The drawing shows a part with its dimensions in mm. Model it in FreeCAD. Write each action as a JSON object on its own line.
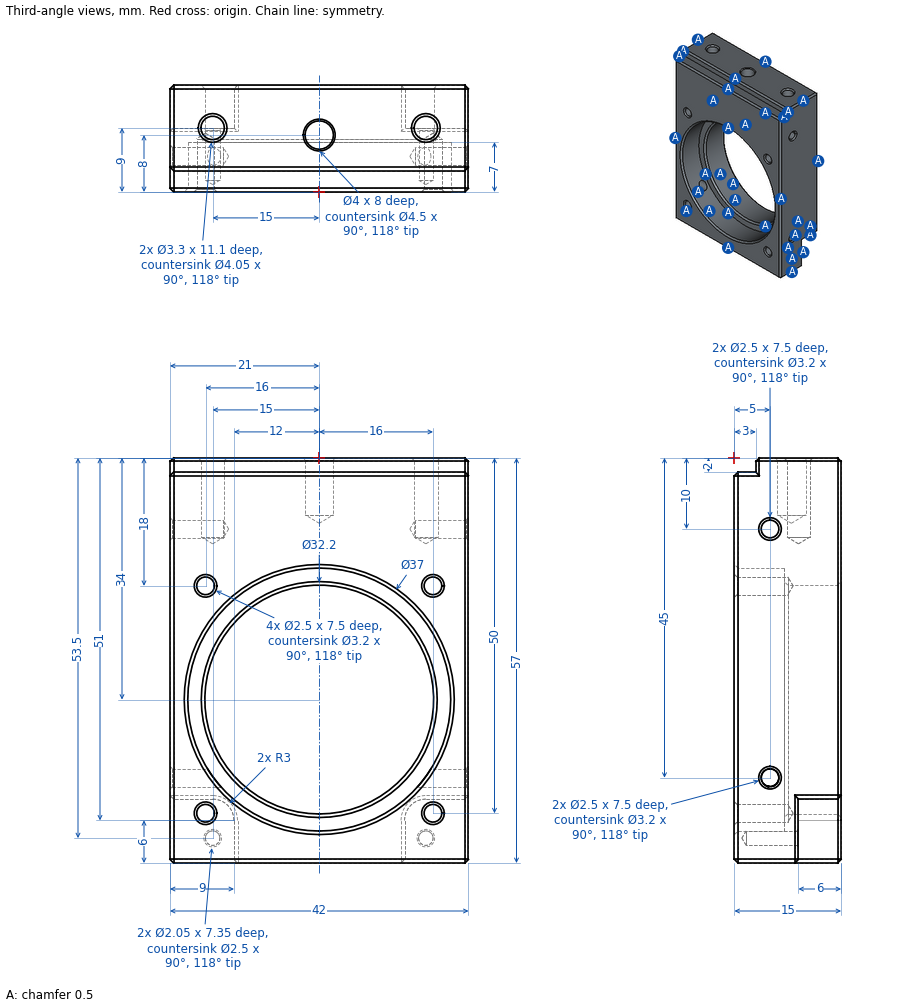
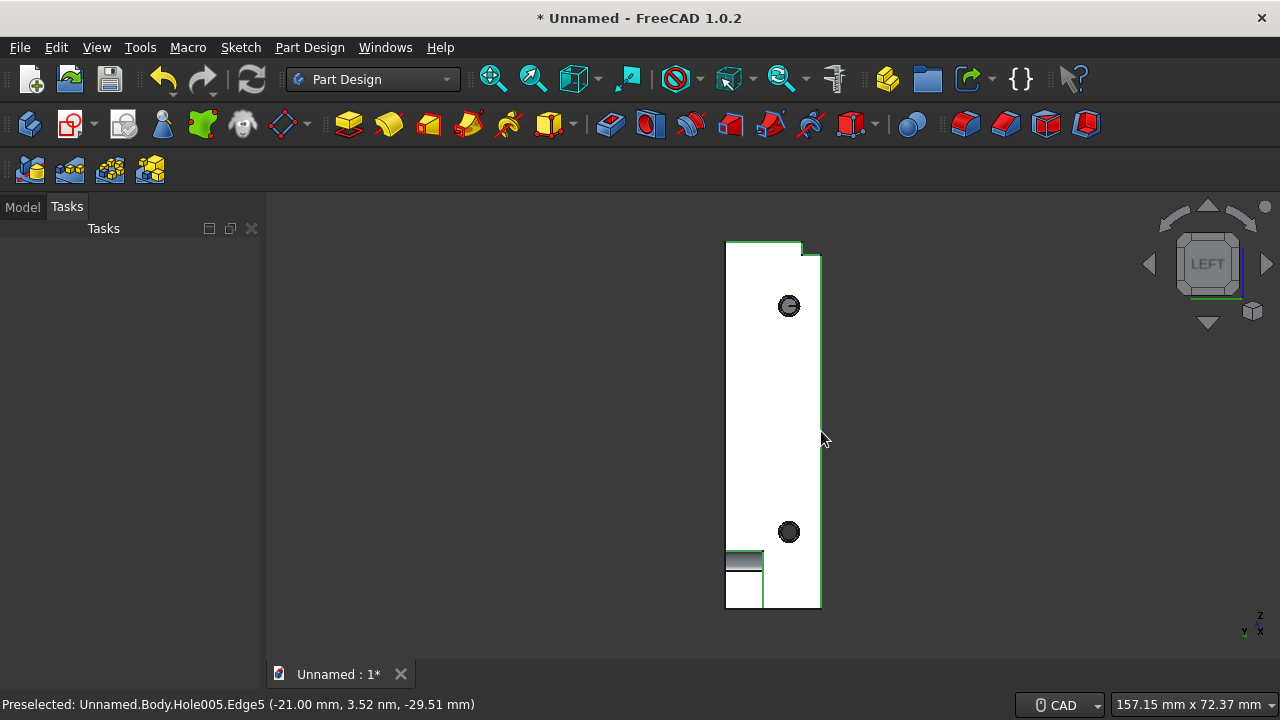
{"action": "left_click", "coordinate": [1006, 124]}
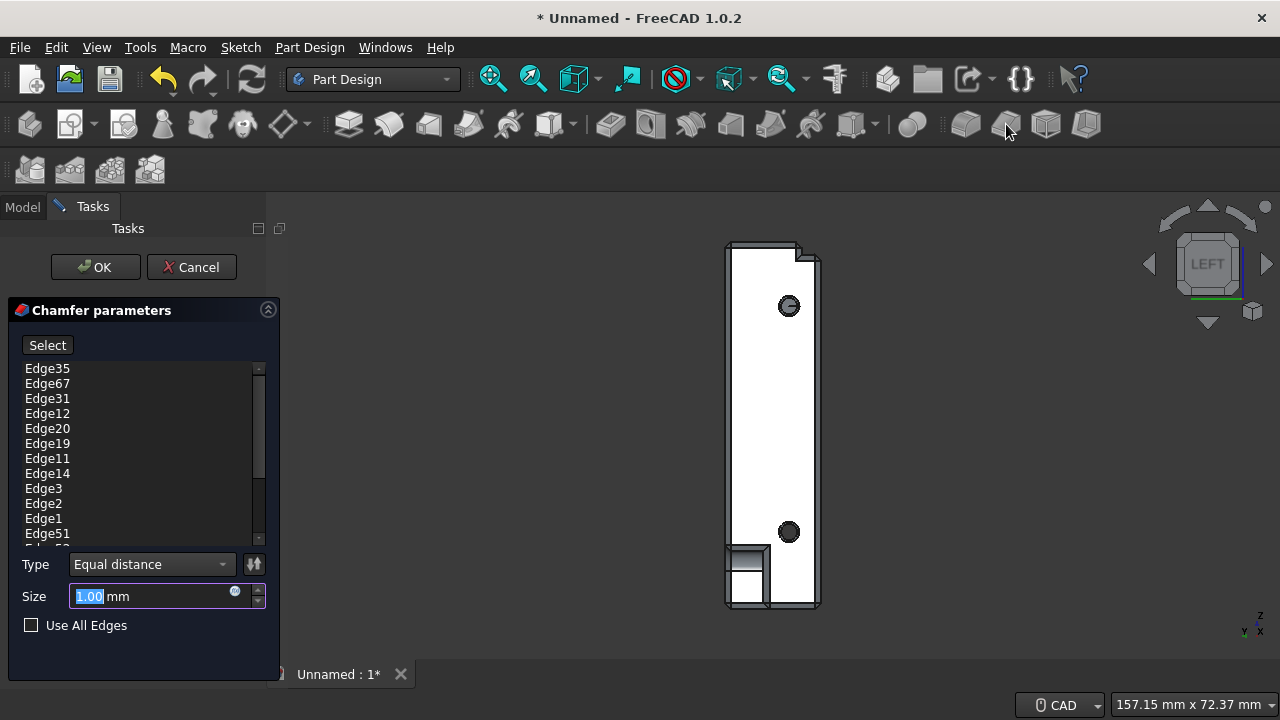
{"action": "type", "text": "0.5"}
{"action": "key", "text": "Tab"}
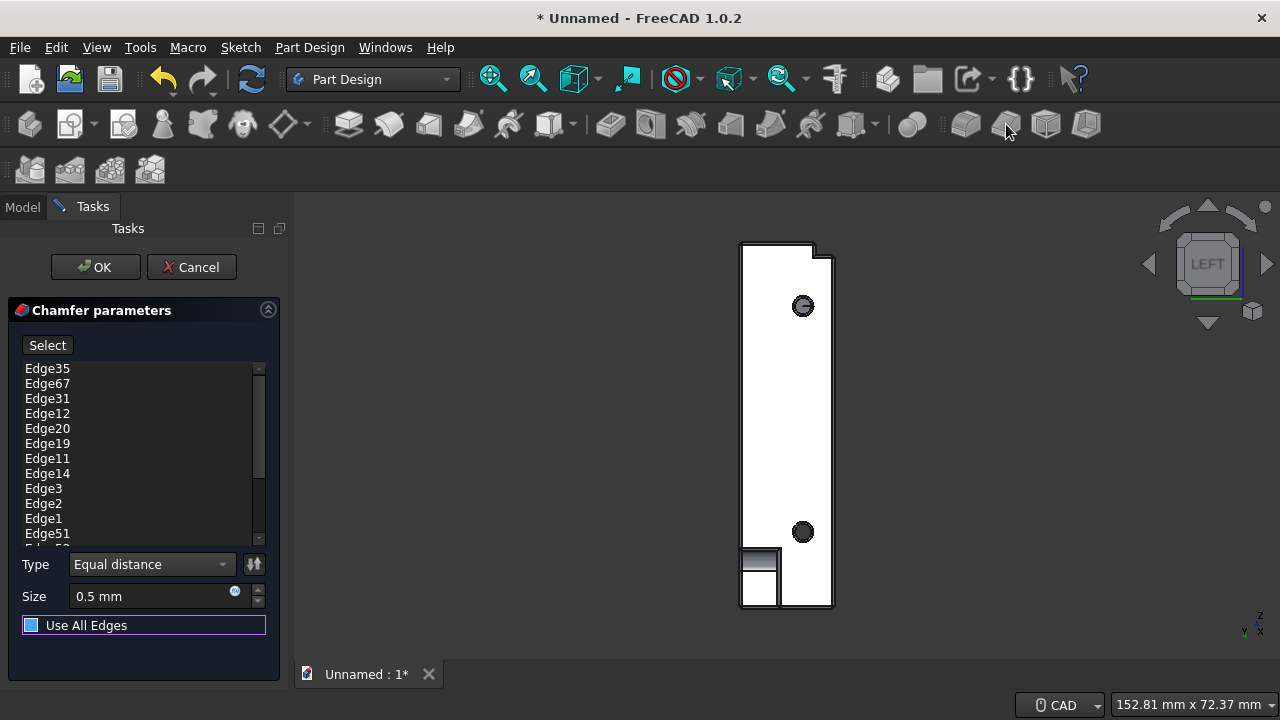
{"action": "left_click", "coordinate": [96, 267]}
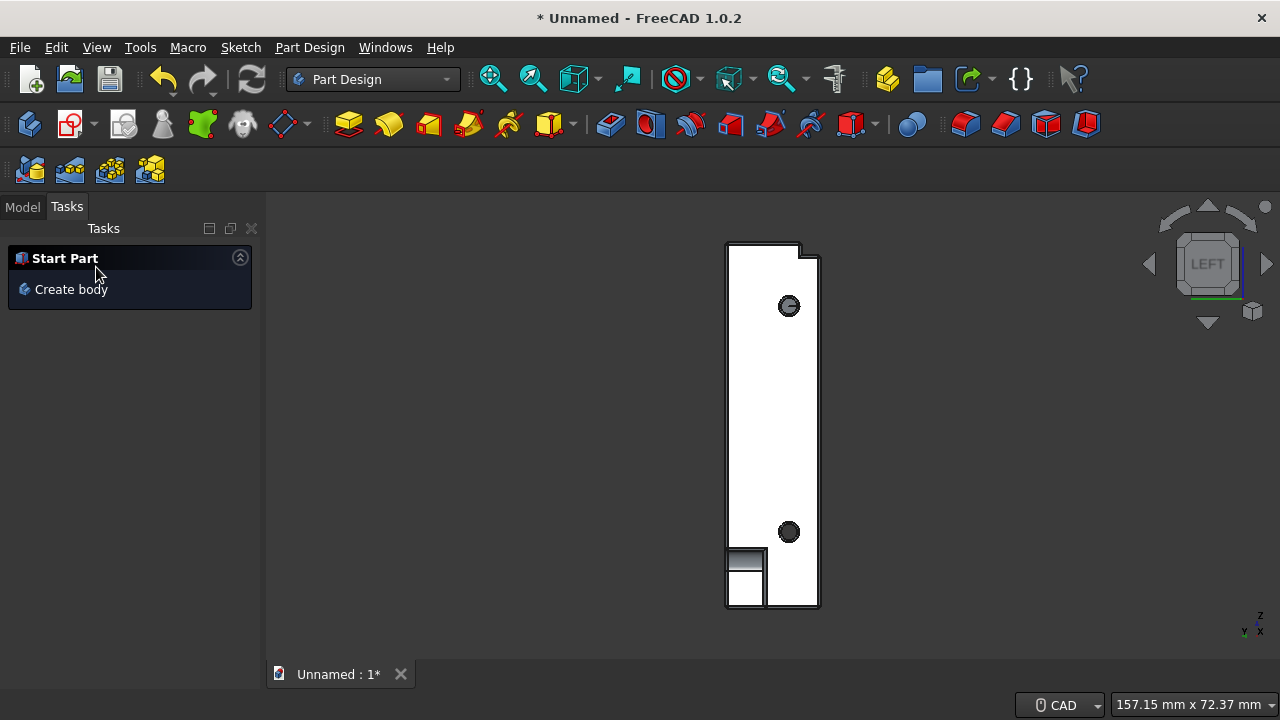
{"action": "key", "text": "0"}